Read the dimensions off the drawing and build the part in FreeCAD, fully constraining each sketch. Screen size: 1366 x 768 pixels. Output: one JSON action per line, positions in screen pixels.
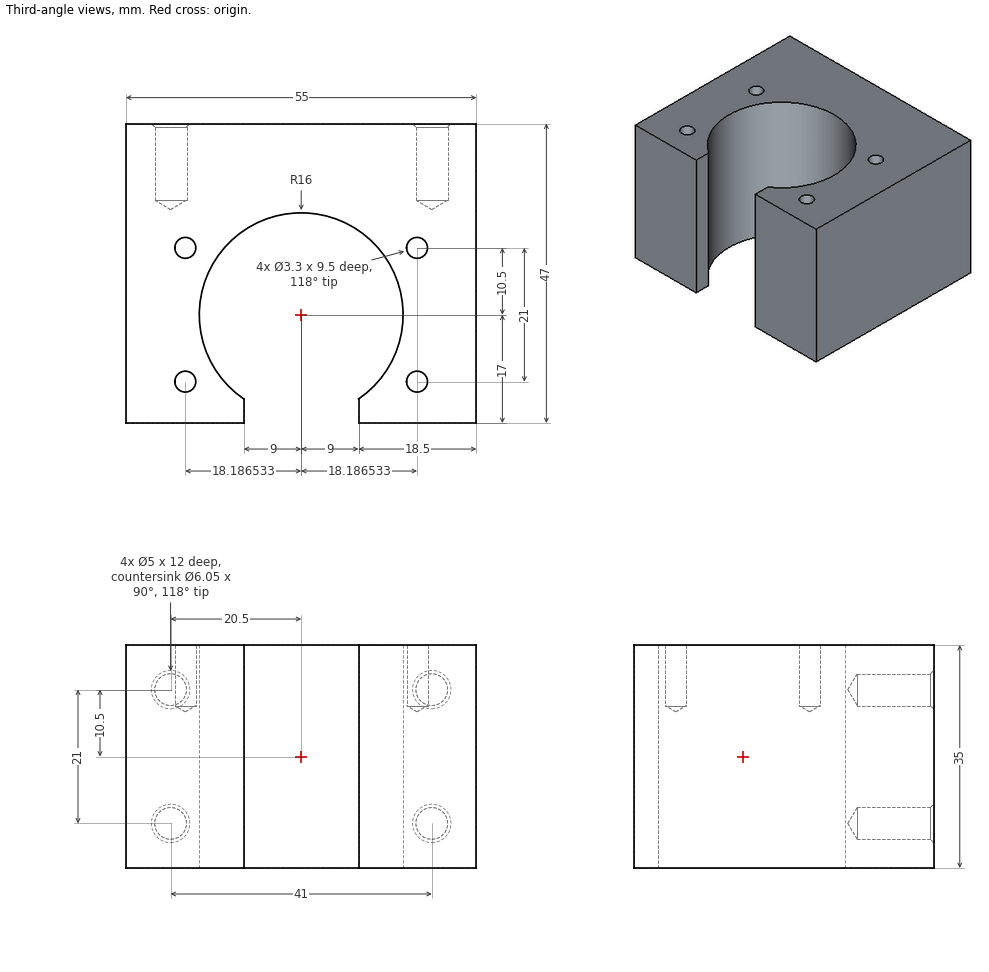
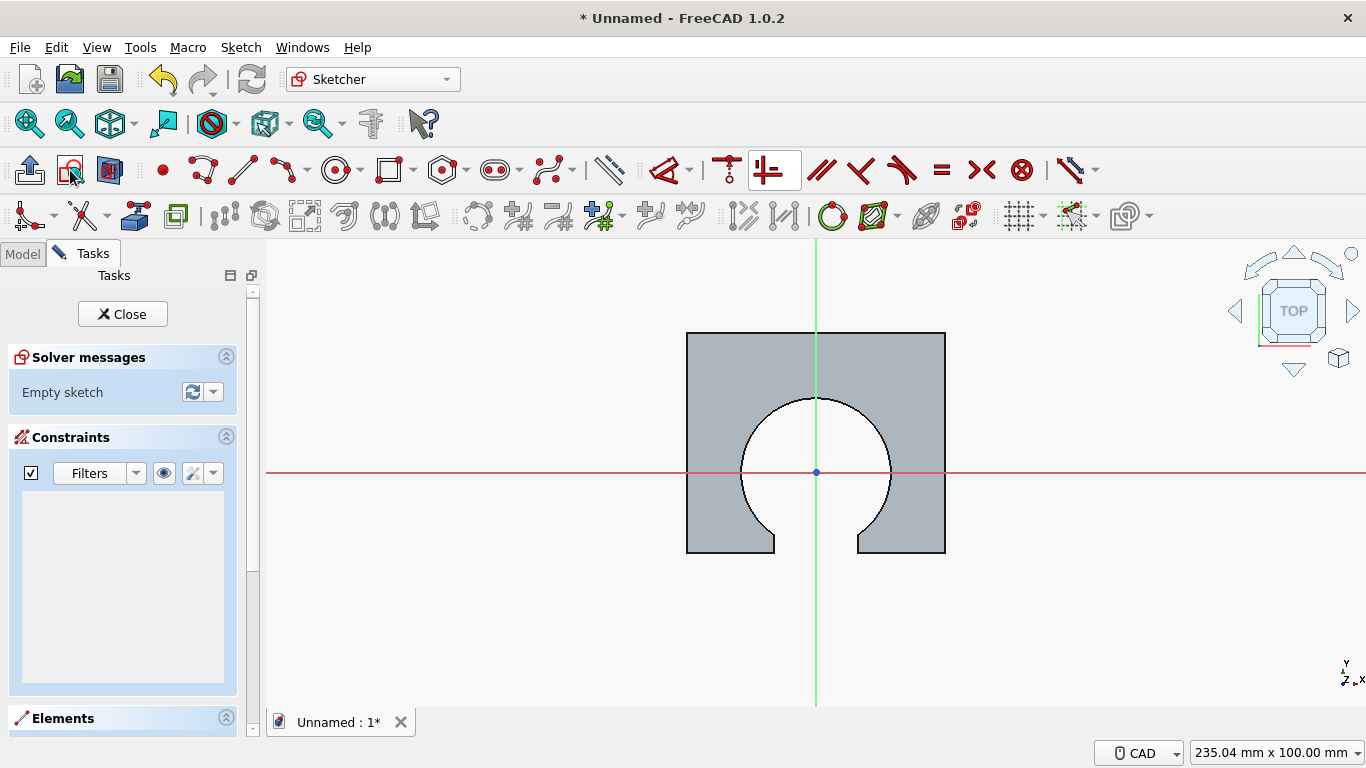
{"action": "scroll", "coordinate": [856, 473], "scroll_direction": "up", "scroll_amount": 5}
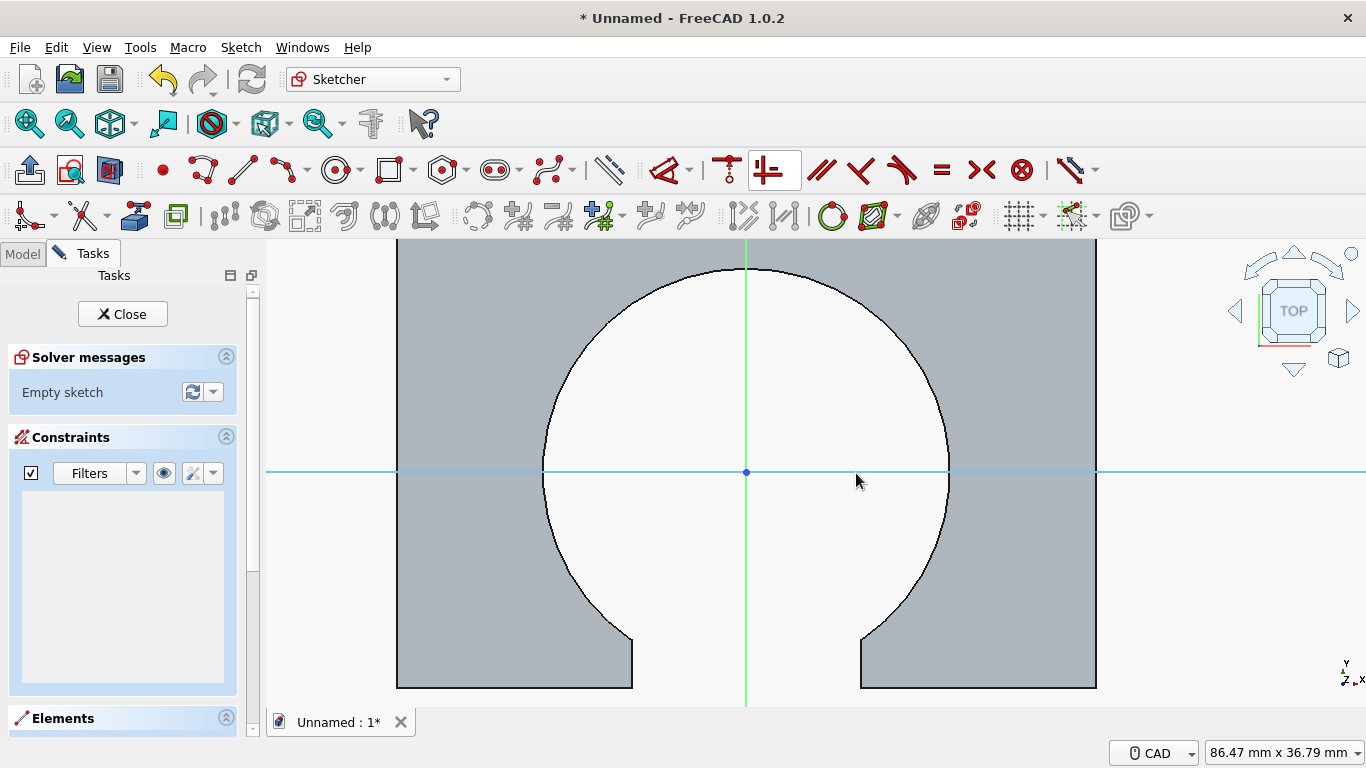
{"action": "left_click", "coordinate": [336, 170]}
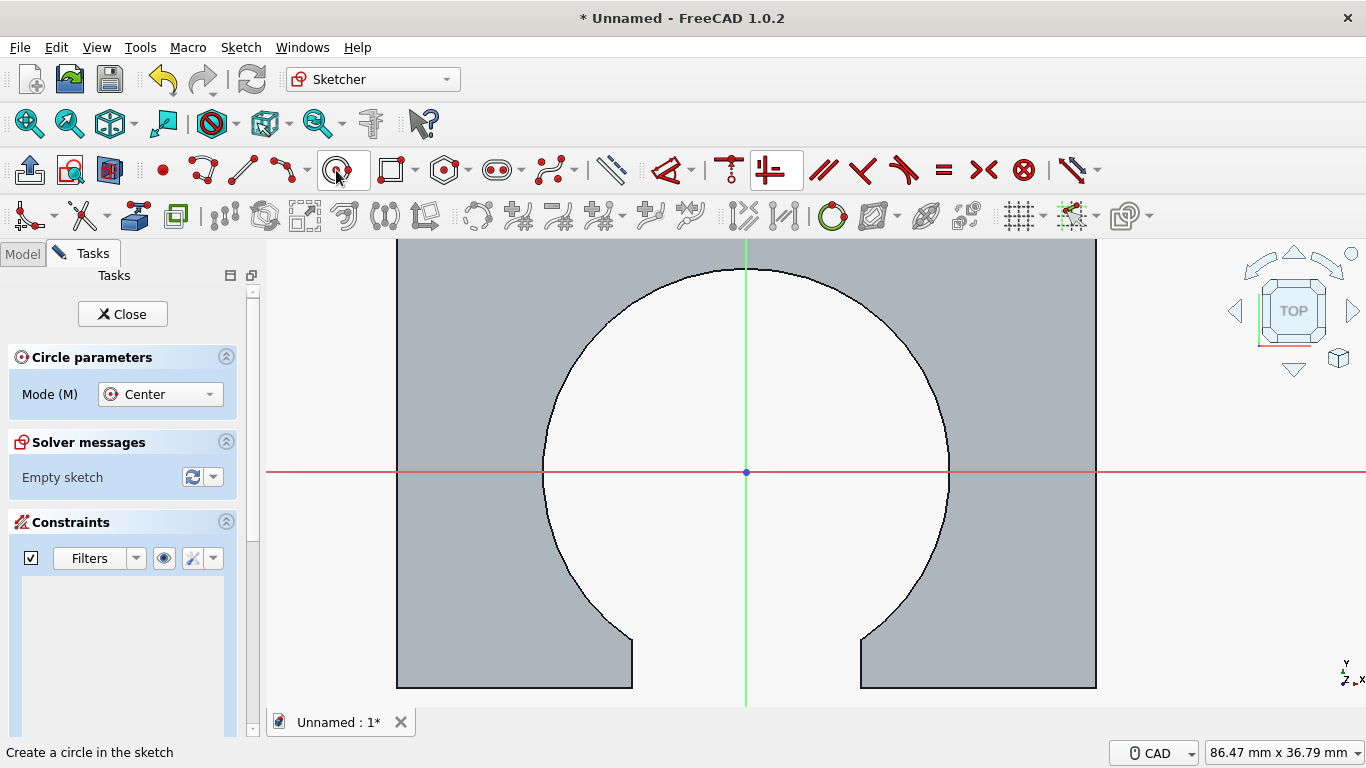
{"action": "left_click", "coordinate": [978, 339]}
{"action": "mouse_move", "coordinate": [993, 324]}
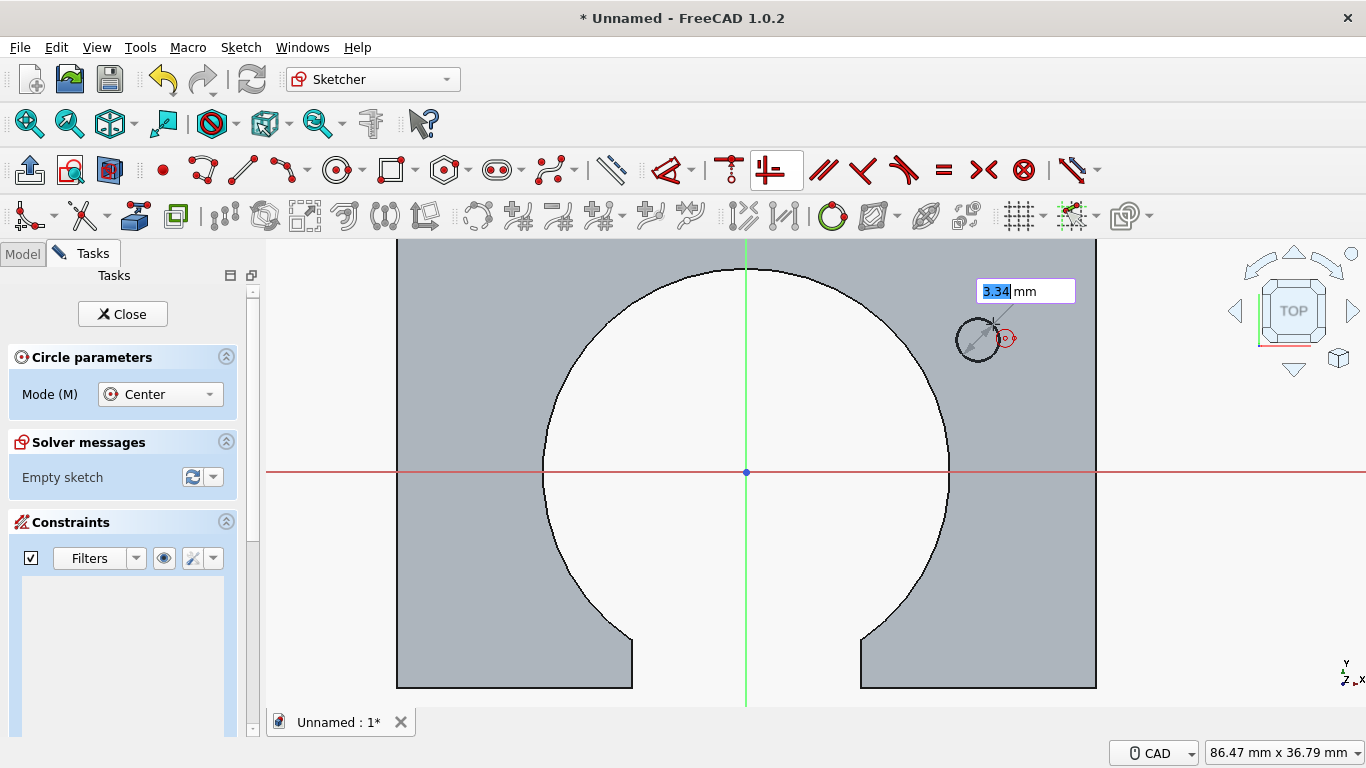
{"action": "type", "text": "3.3"}
{"action": "key", "text": "Return"}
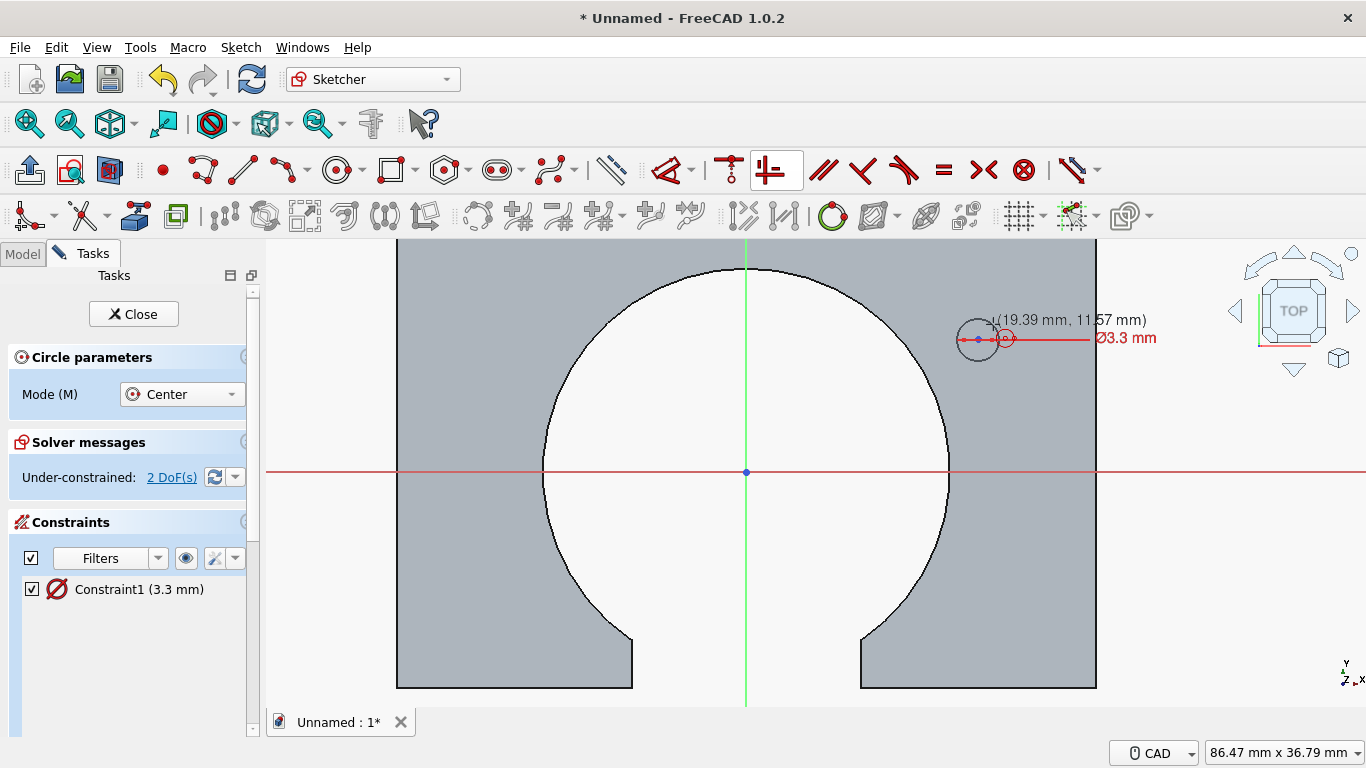
{"action": "left_click", "coordinate": [978, 606]}
{"action": "mouse_move", "coordinate": [993, 591]}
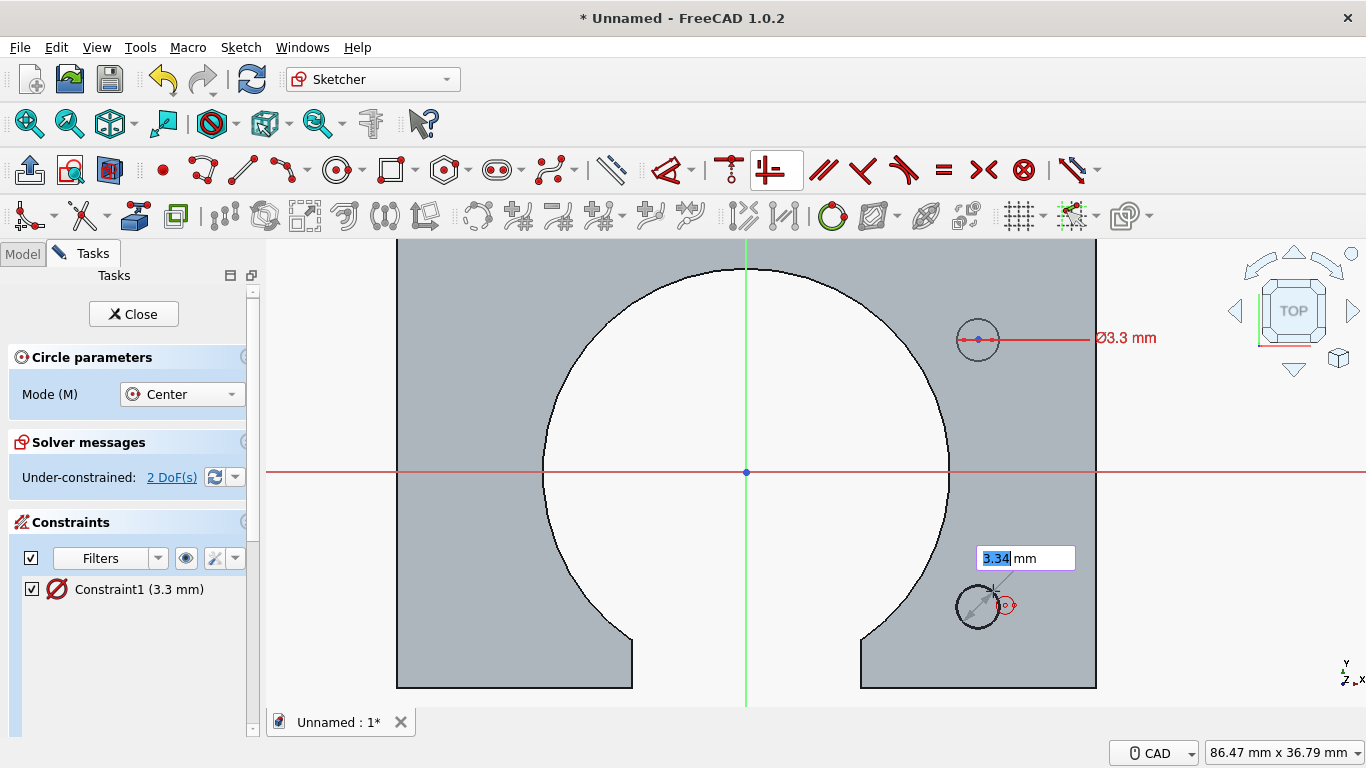
{"action": "type", "text": "3.3"}
{"action": "key", "text": "Return"}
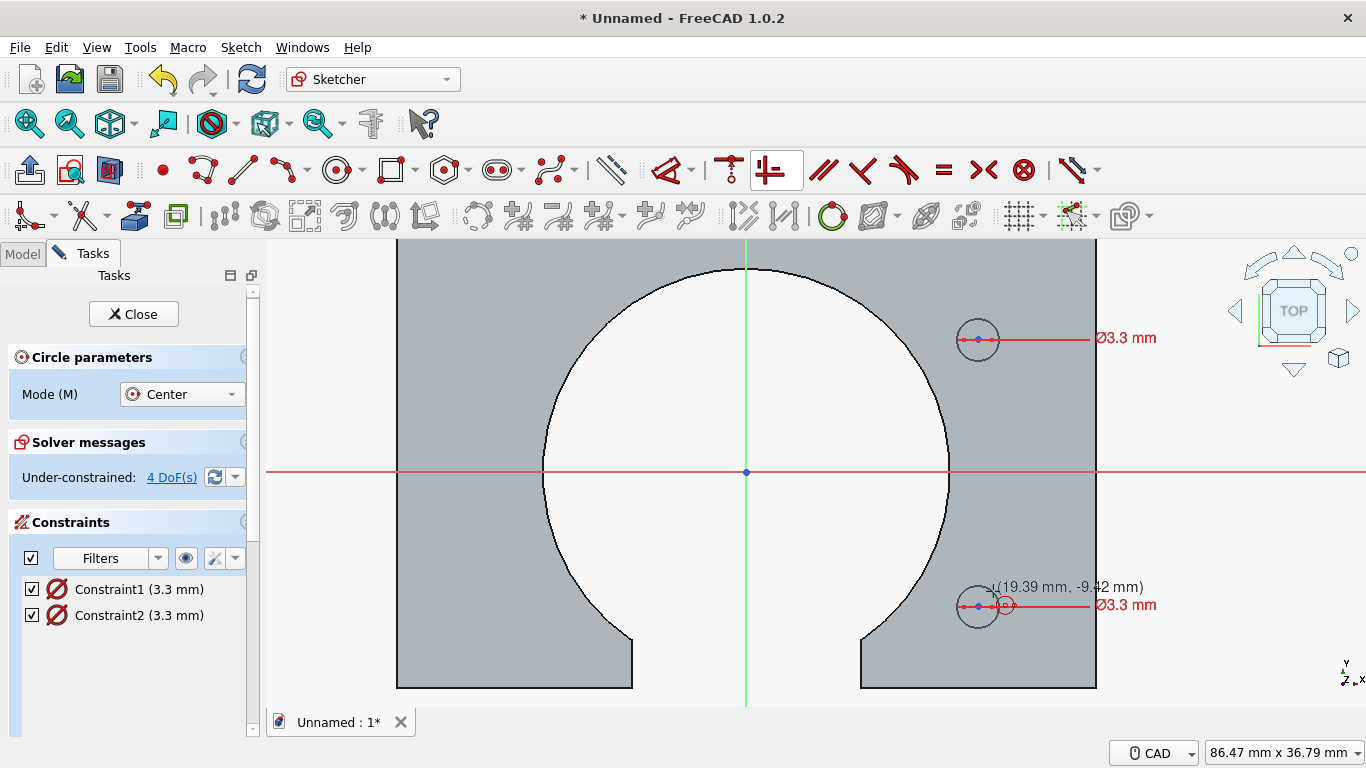
{"action": "left_click", "coordinate": [515, 606]}
{"action": "mouse_move", "coordinate": [530, 591]}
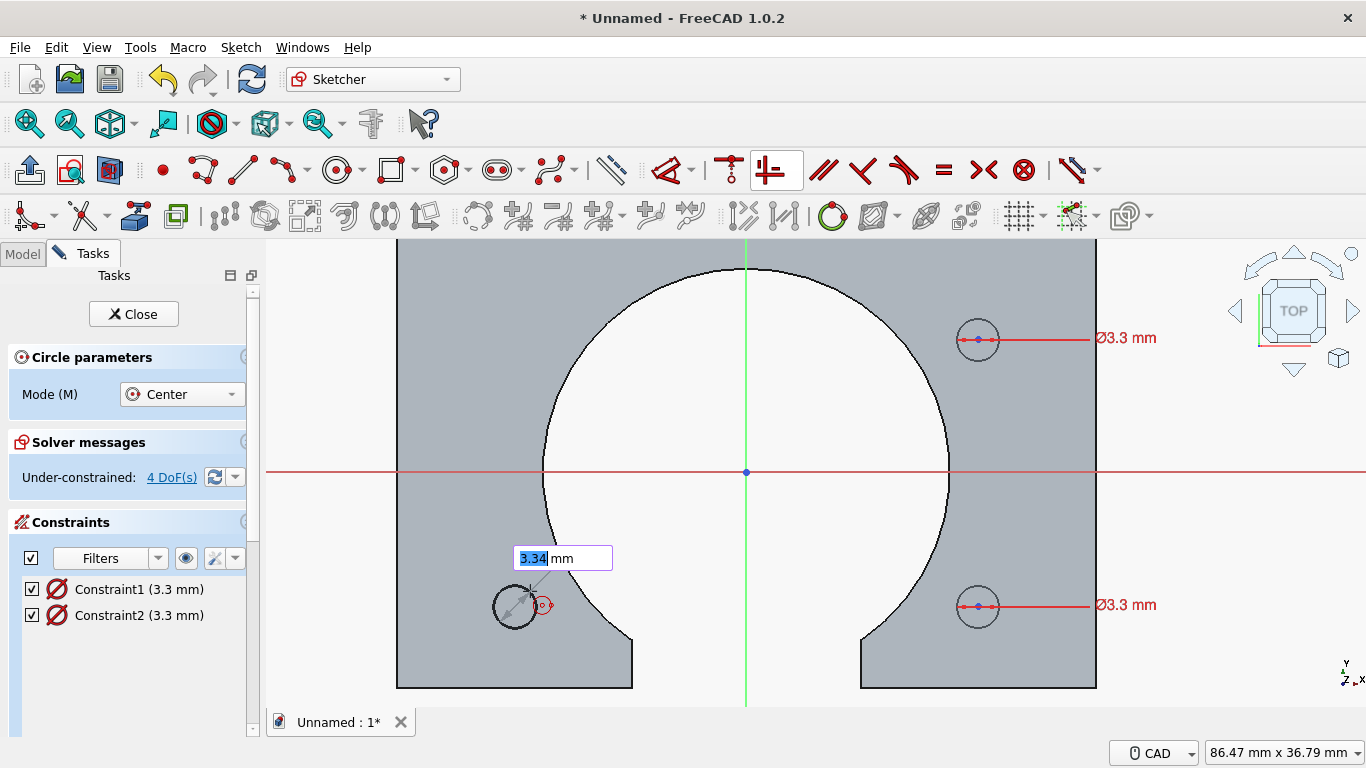
{"action": "type", "text": "3.3"}
{"action": "key", "text": "Return"}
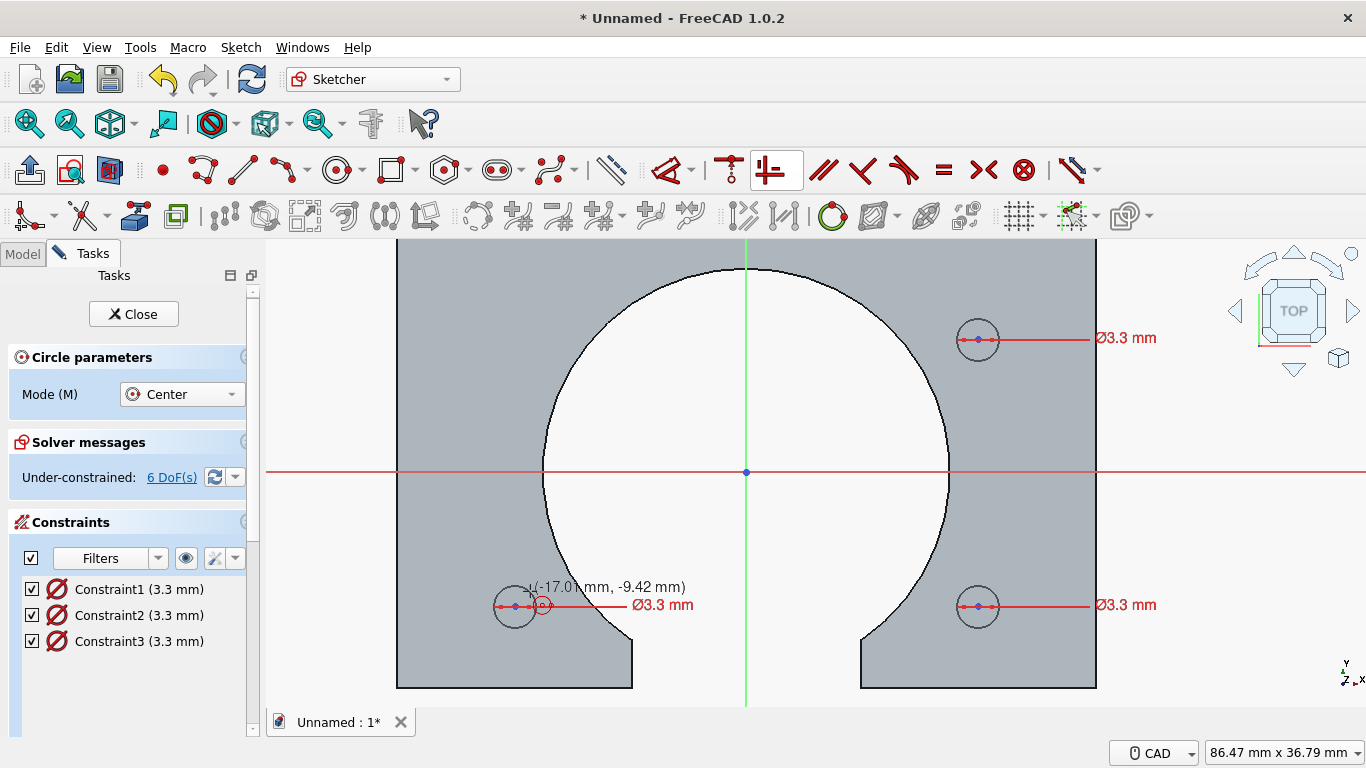
{"action": "left_click", "coordinate": [515, 339]}
{"action": "mouse_move", "coordinate": [530, 324]}